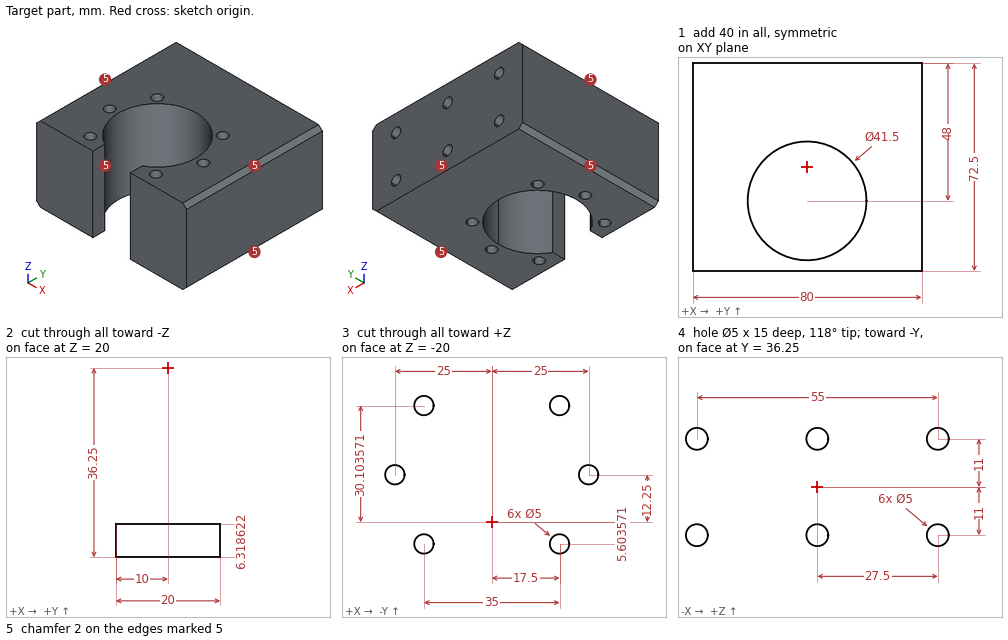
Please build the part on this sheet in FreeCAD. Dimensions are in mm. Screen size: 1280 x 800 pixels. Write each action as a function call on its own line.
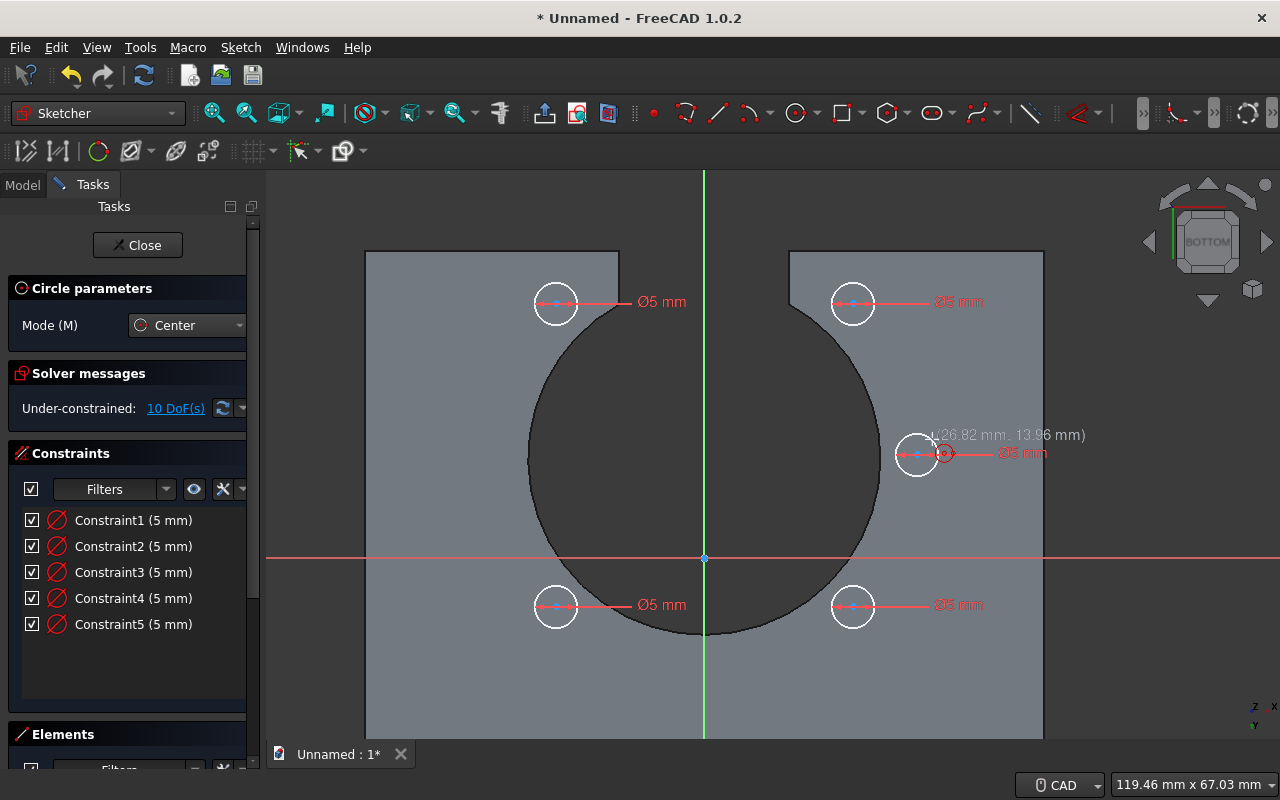
click(492, 454)
move(507, 439)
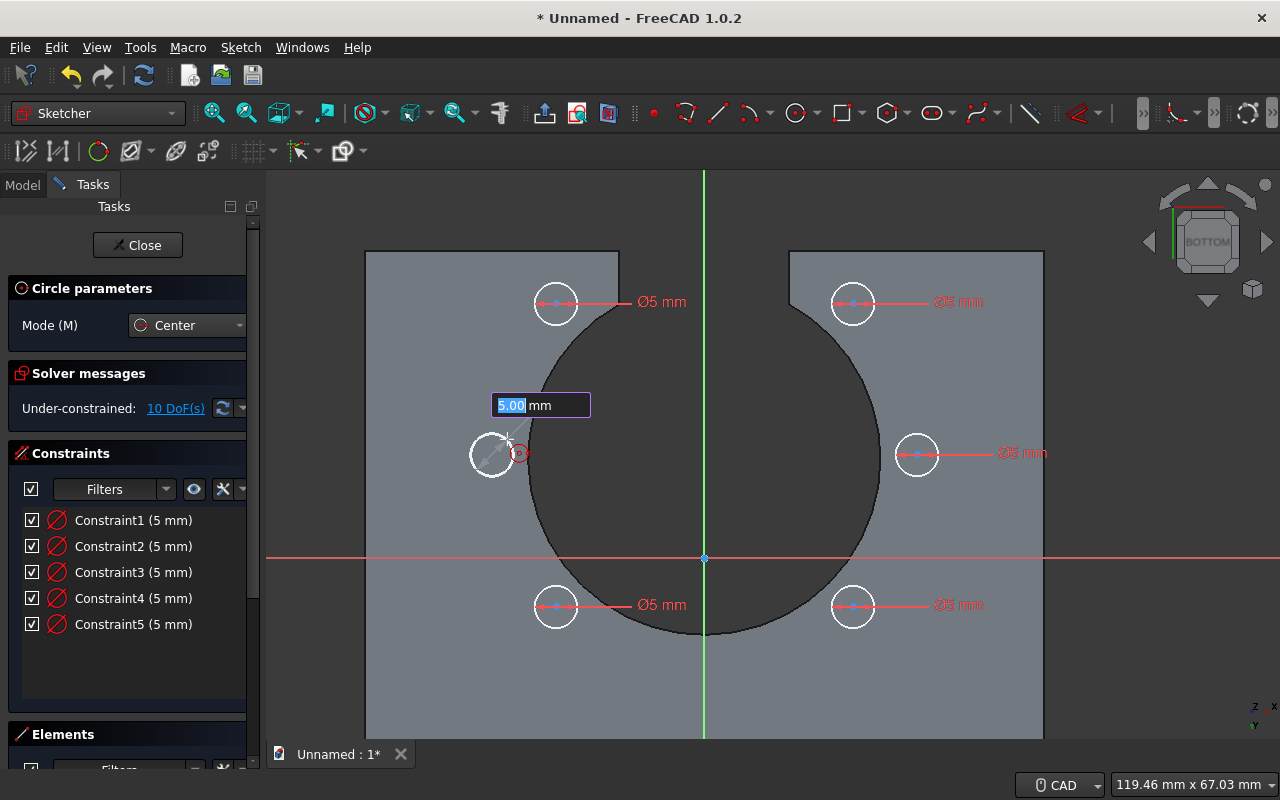
text(5)
key(Return)
key(Escape)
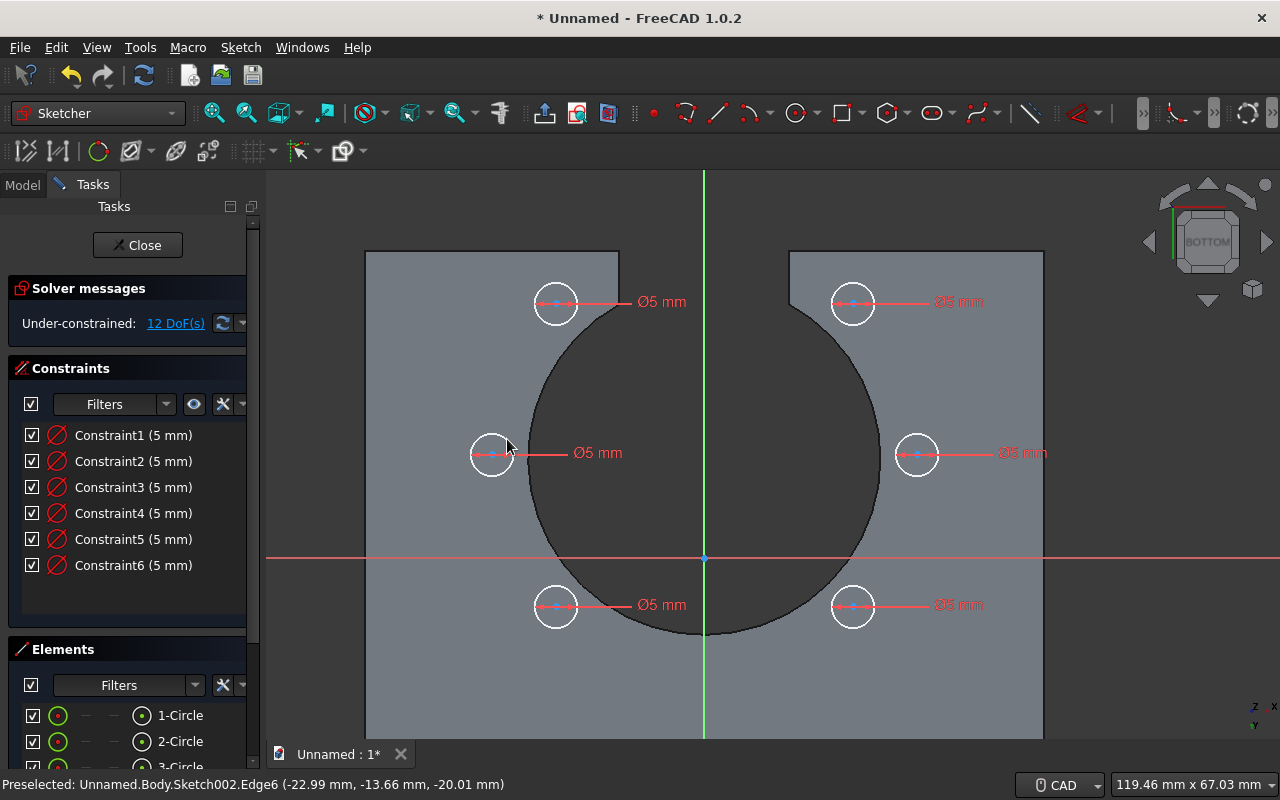
click(853, 607)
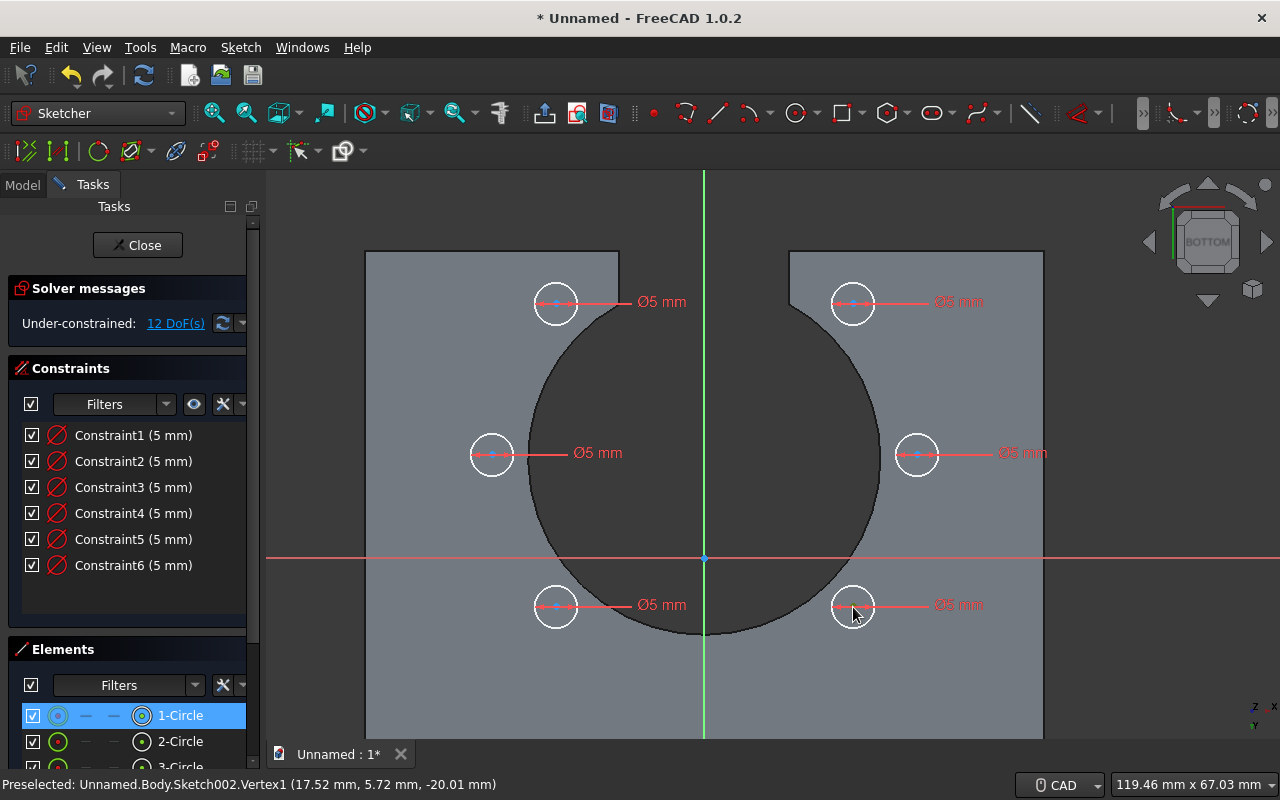
click(556, 607)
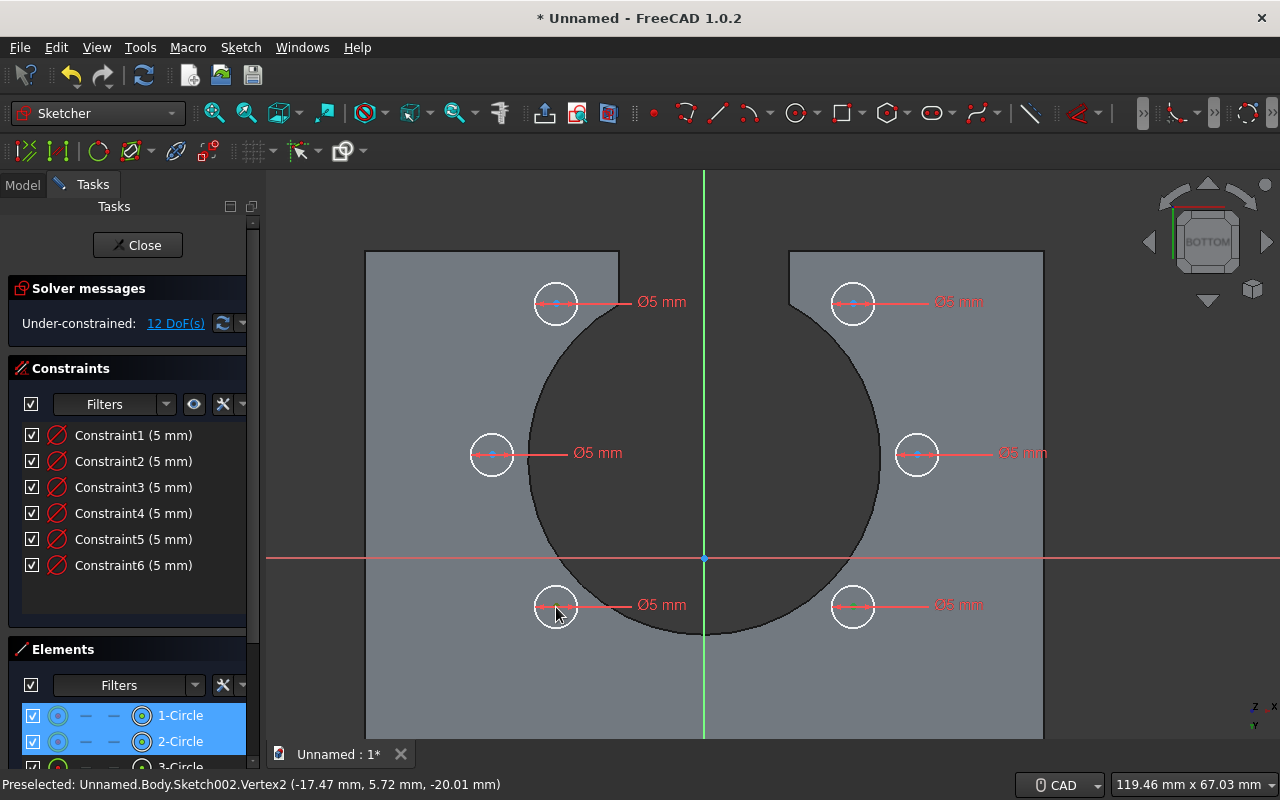
key(h)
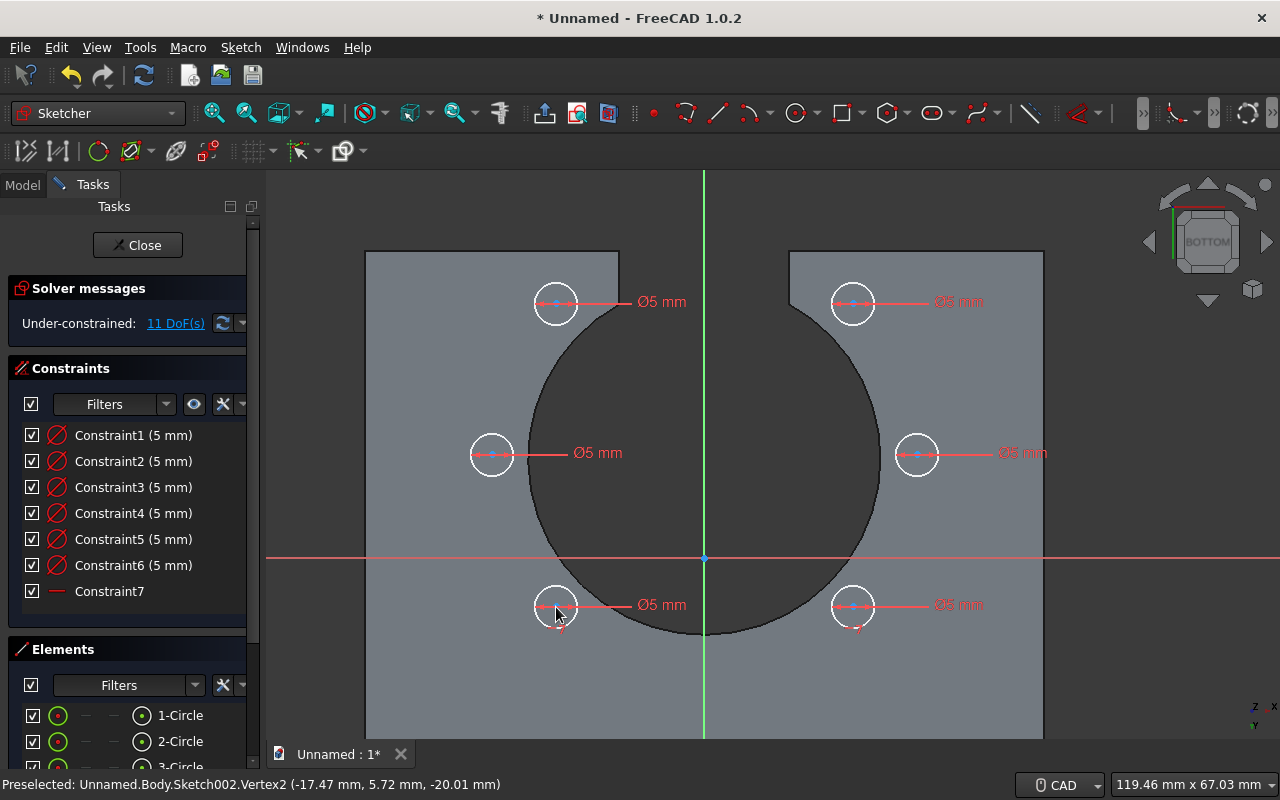
click(556, 607)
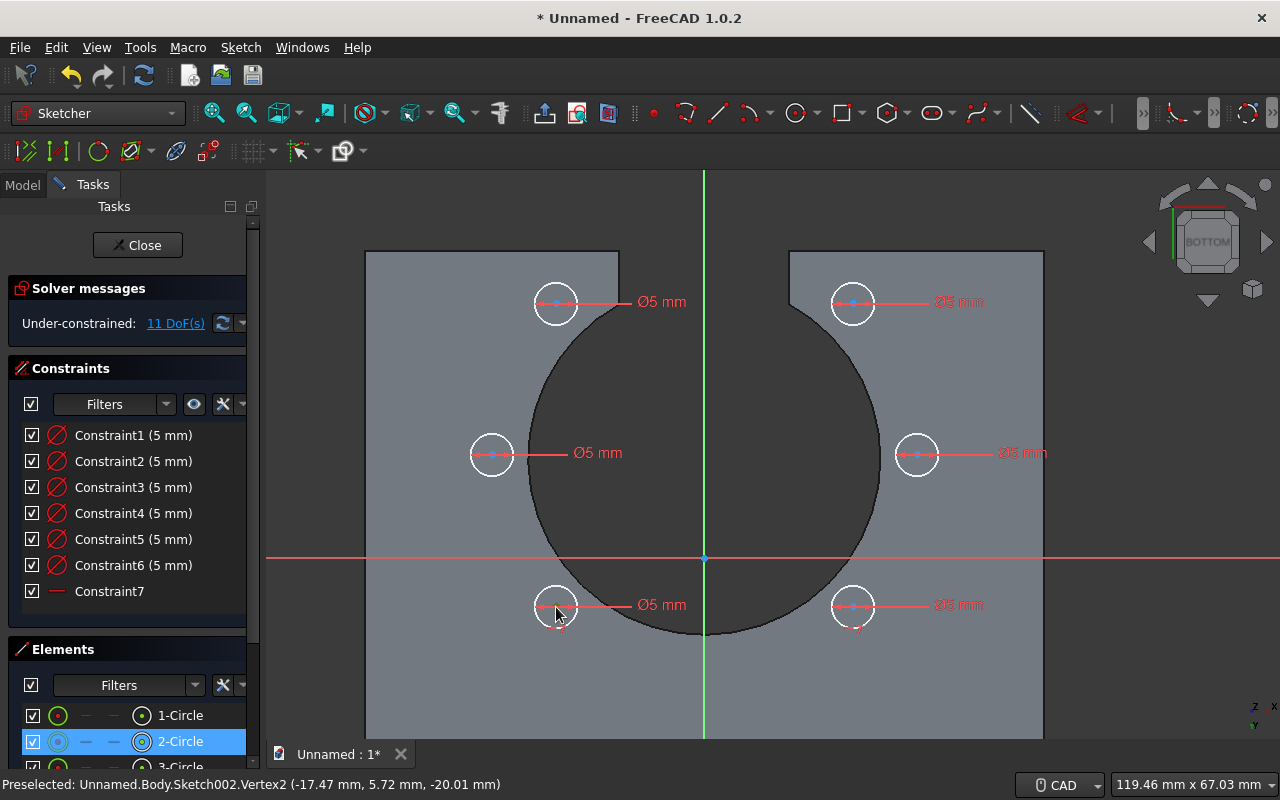
click(556, 304)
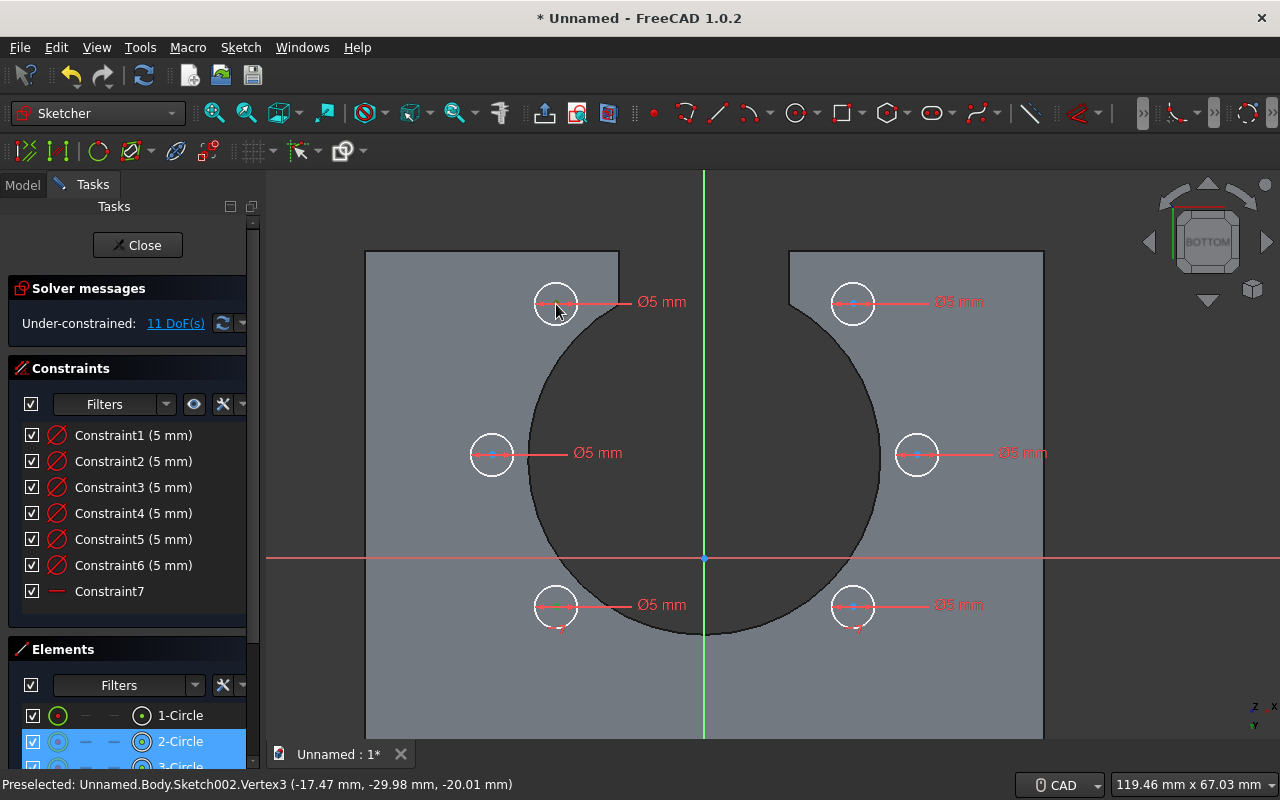
key(v)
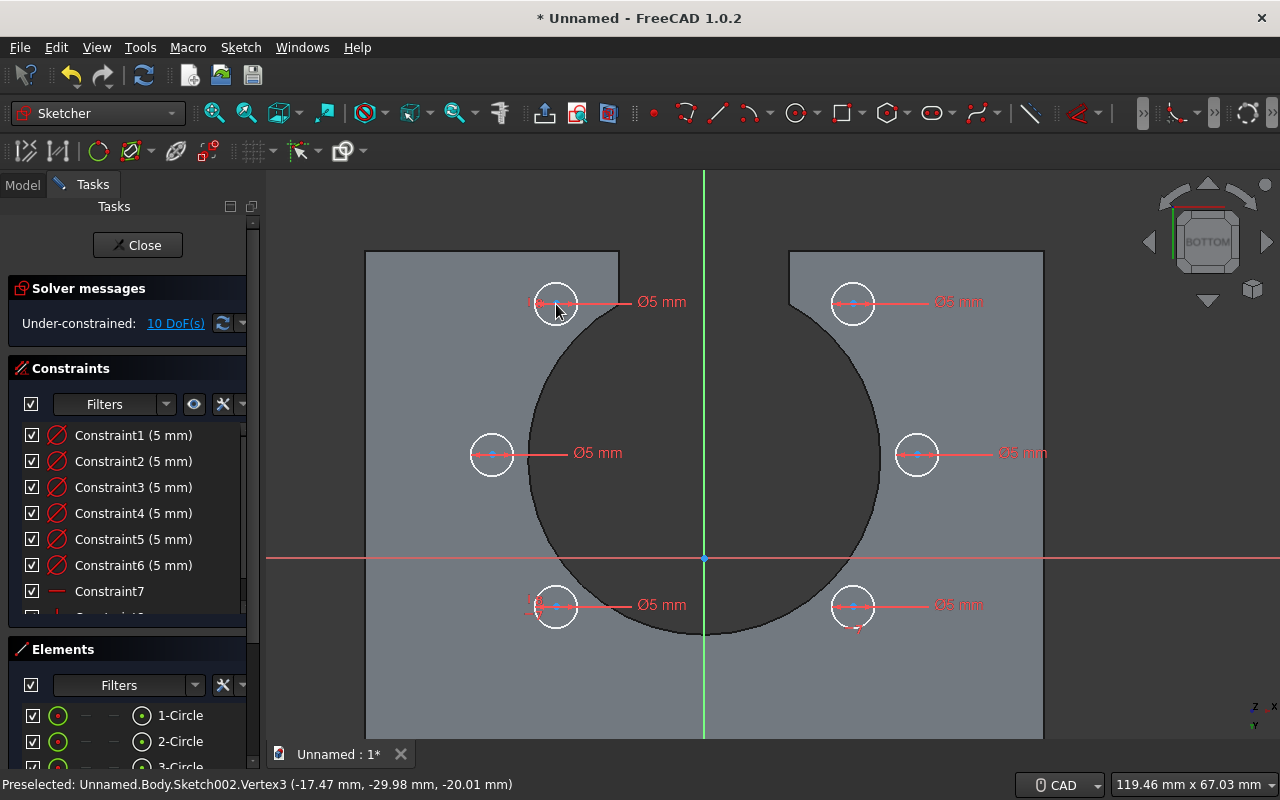
click(853, 607)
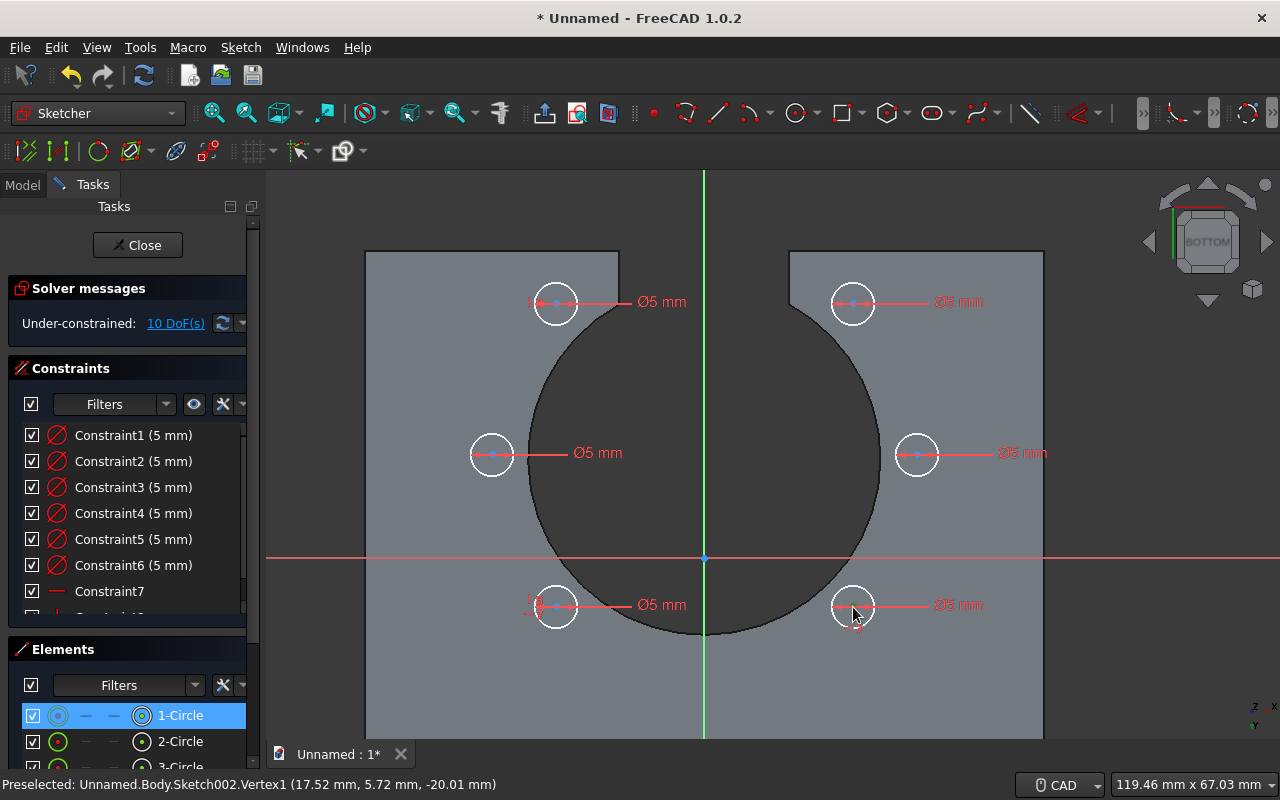
click(853, 304)